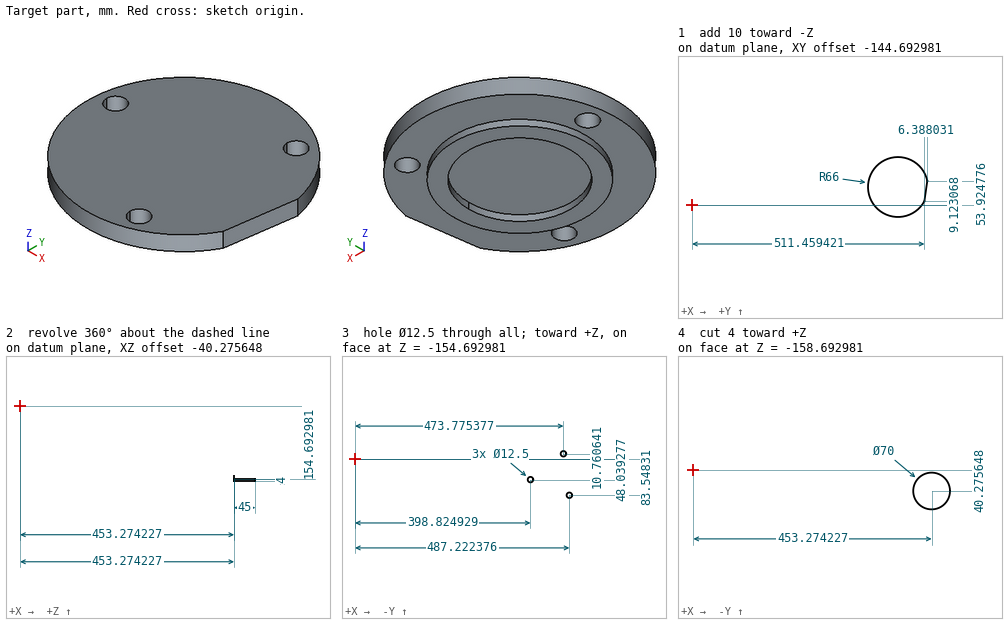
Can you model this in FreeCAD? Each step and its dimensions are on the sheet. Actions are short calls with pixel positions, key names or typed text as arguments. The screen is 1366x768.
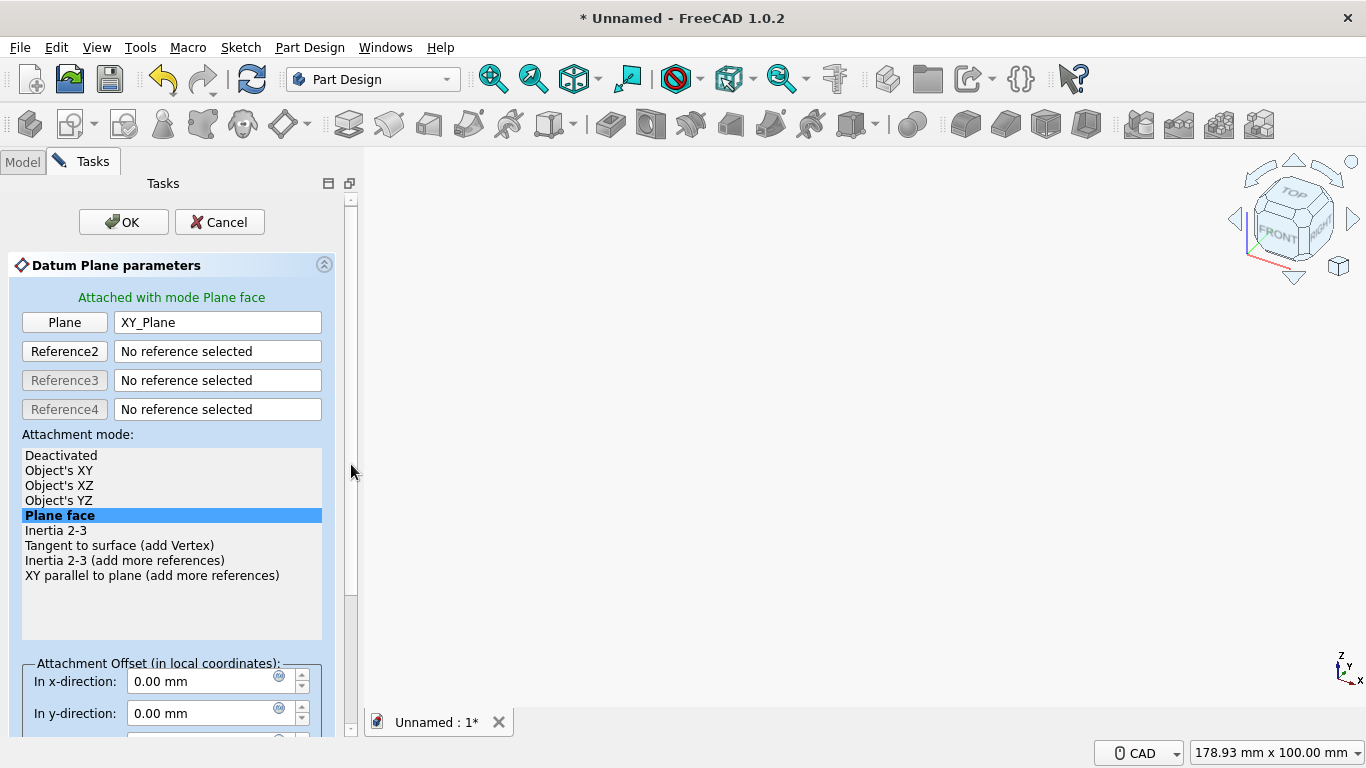
click(124, 222)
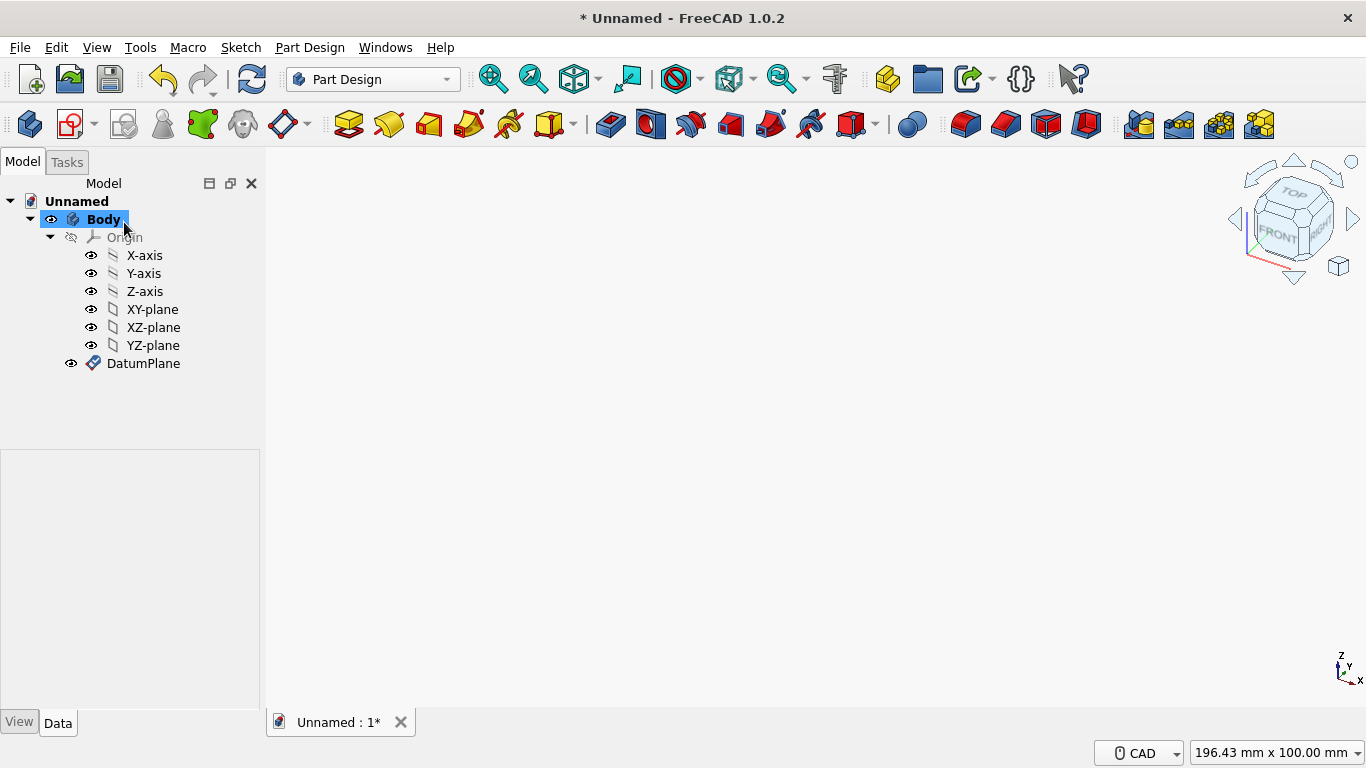
click(116, 363)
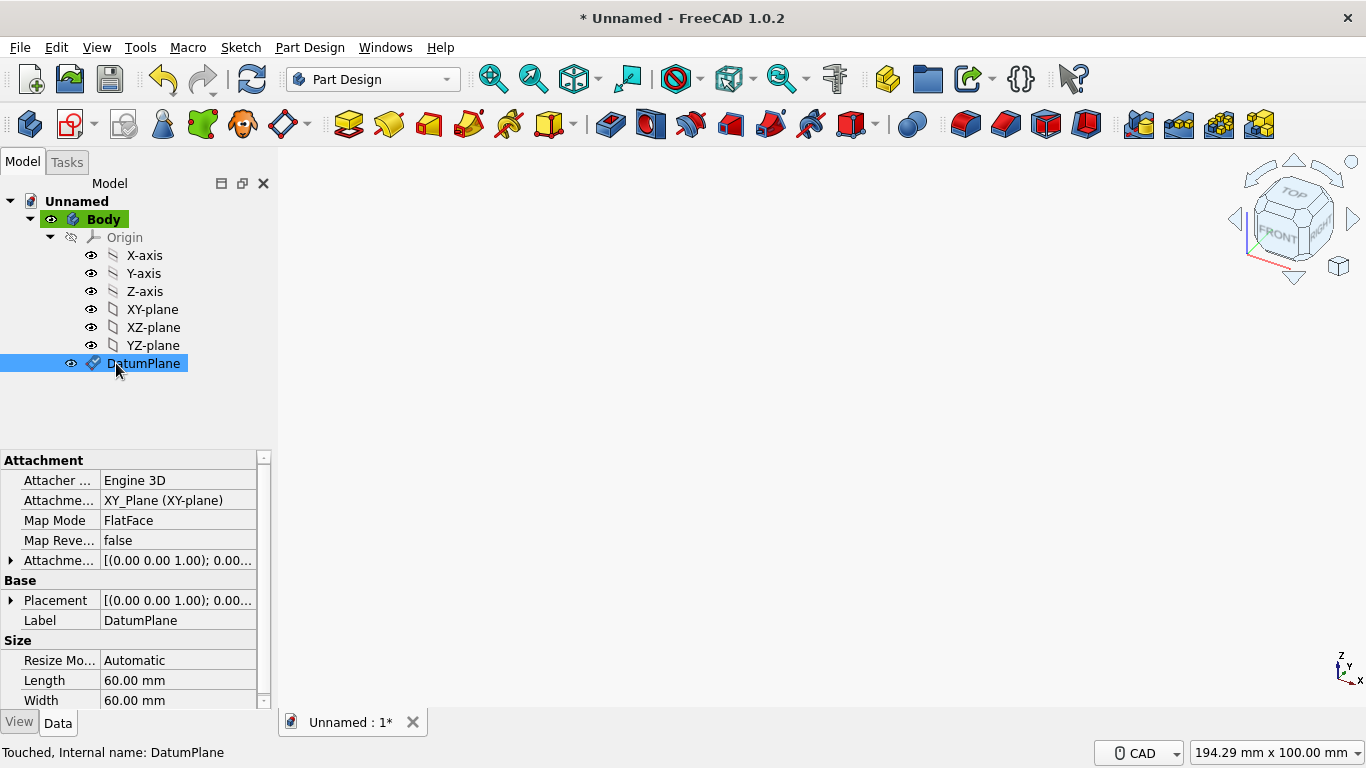
click(70, 124)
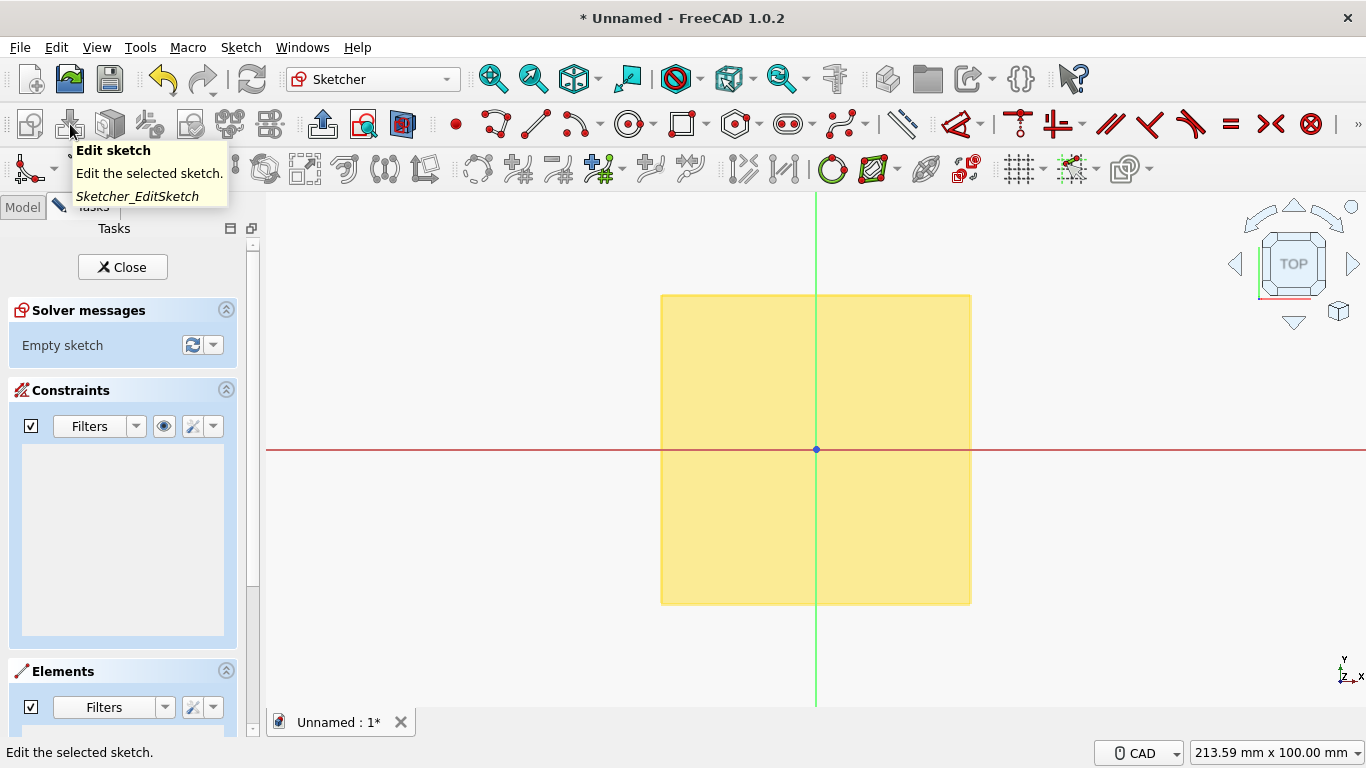
scroll(748, 450, down, 5)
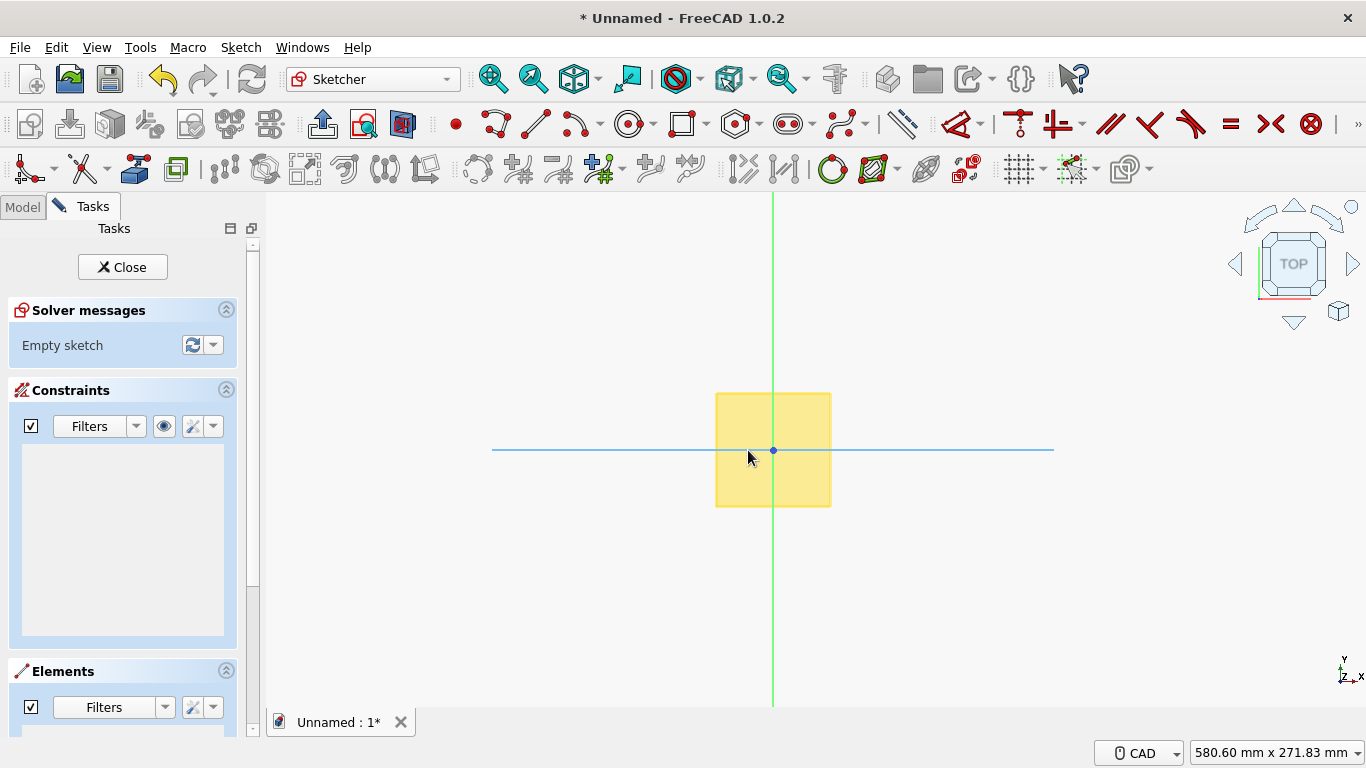
scroll(748, 450, down, 5)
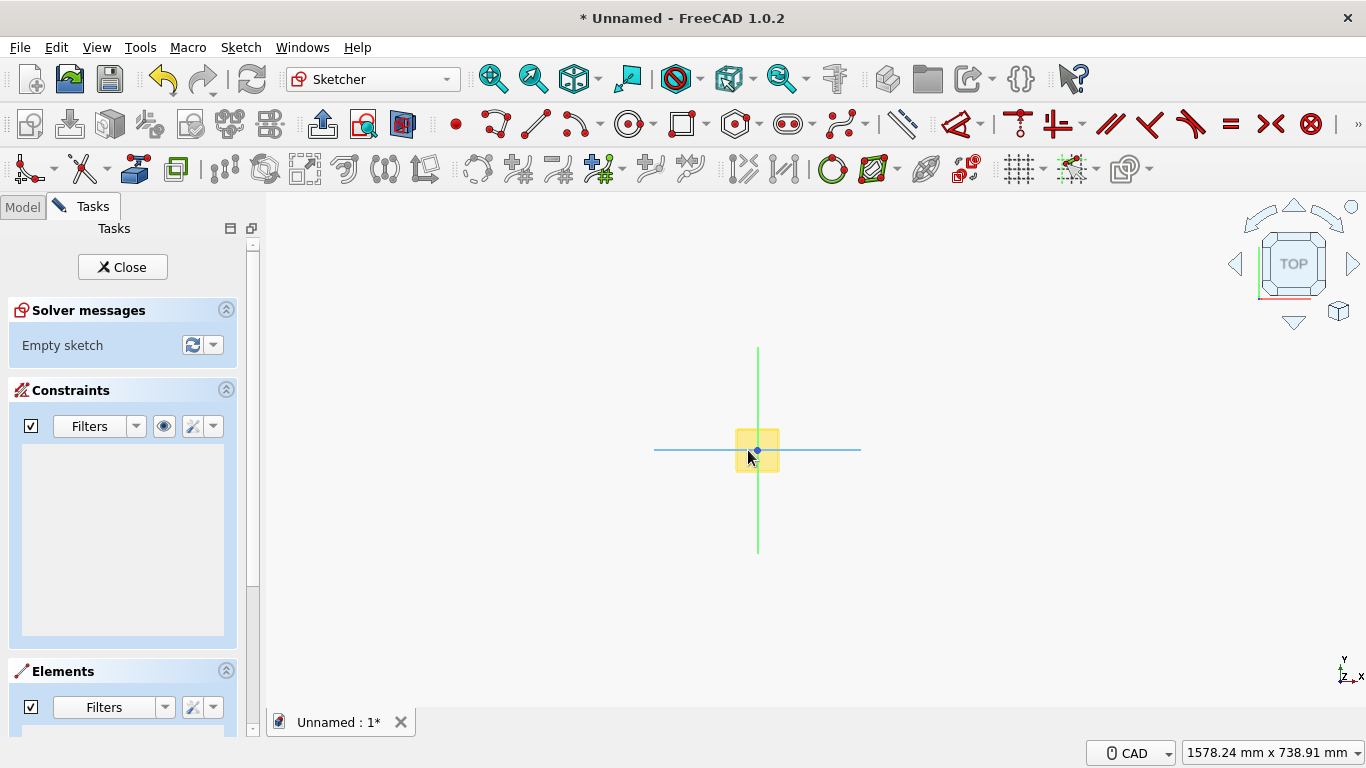
scroll(1124, 425, up, 10)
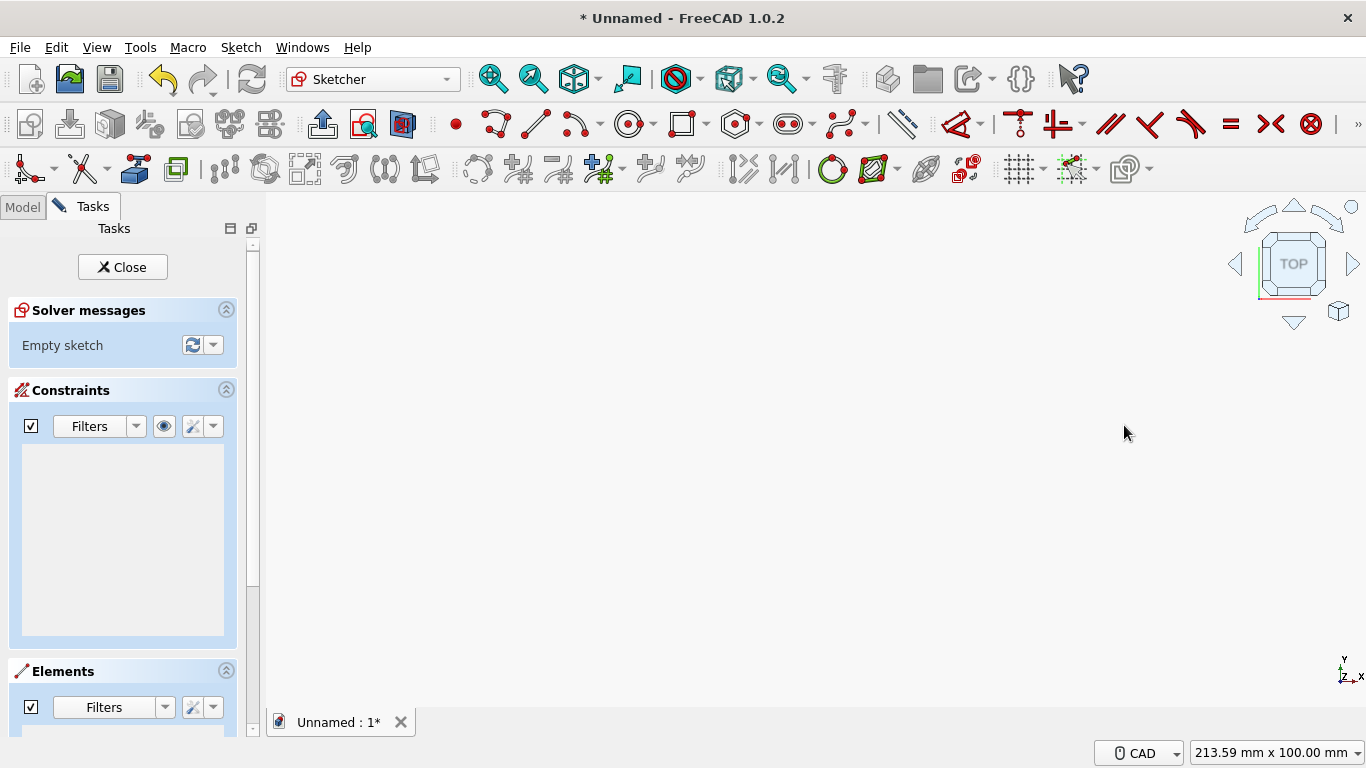
key(g)
key(l)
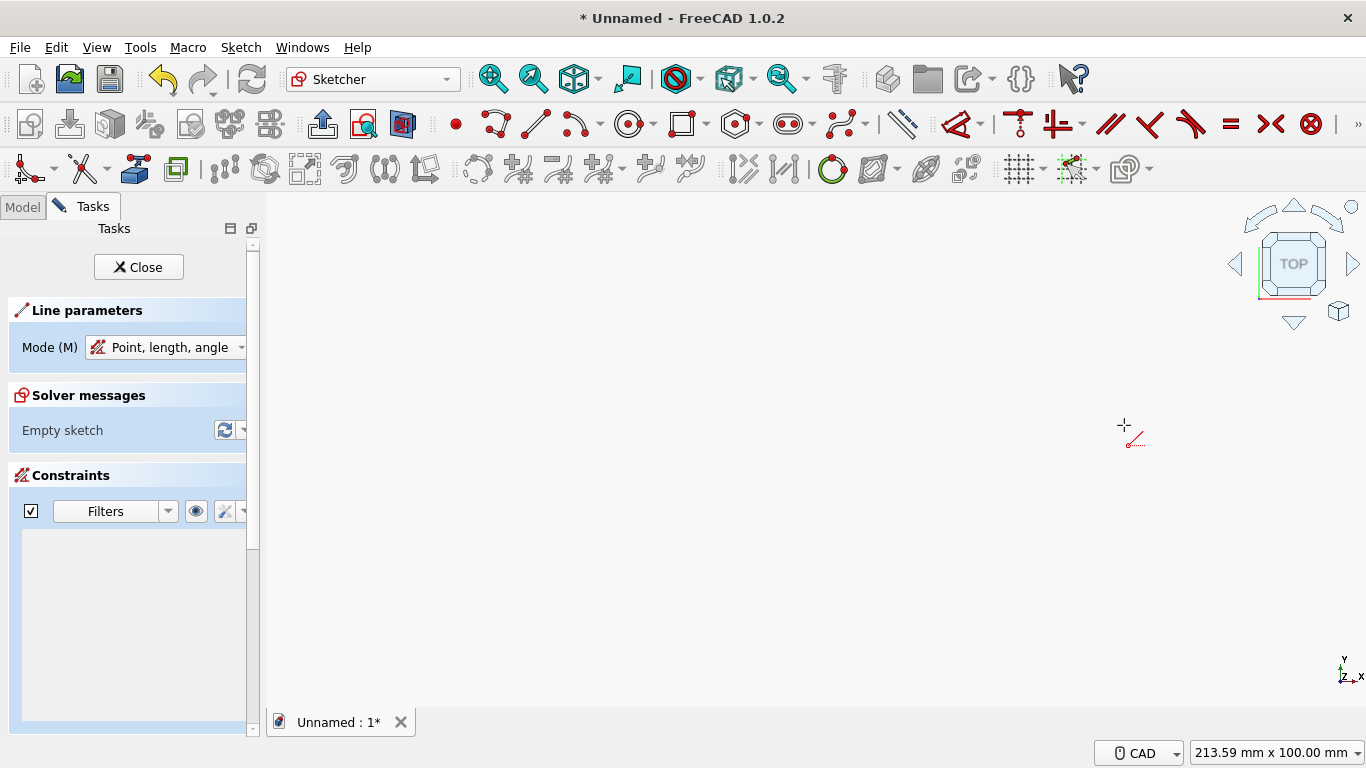
click(1046, 563)
click(1078, 332)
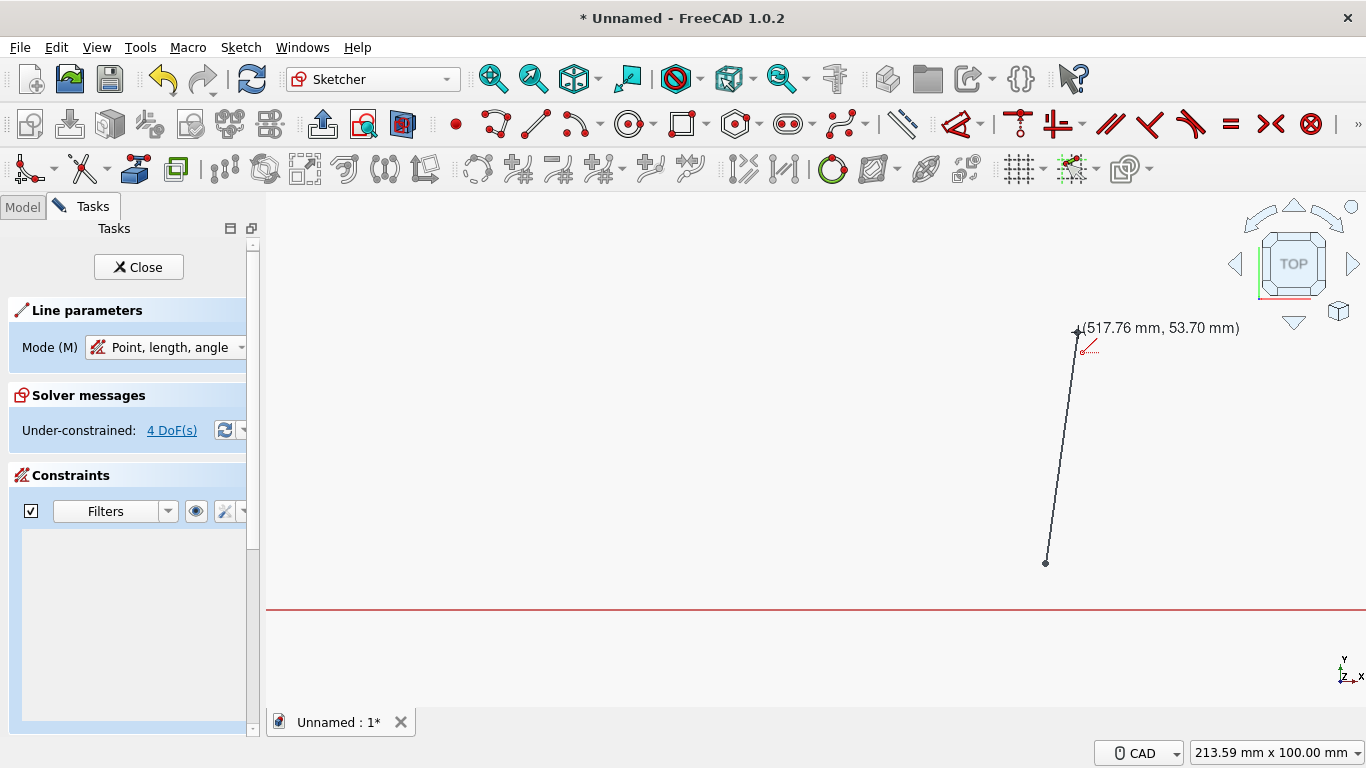
key(g)
key(3)
key(a)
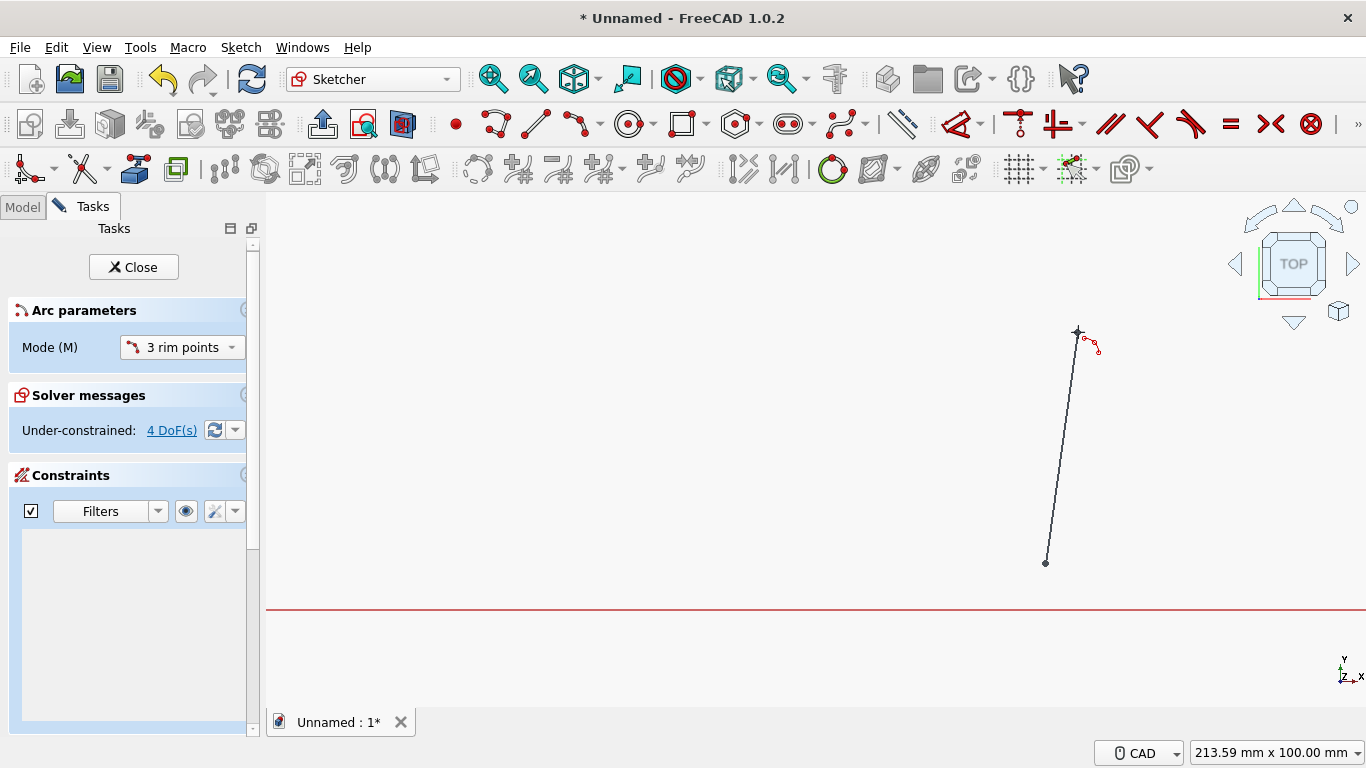
click(1078, 333)
click(1046, 564)
click(409, 354)
key(Escape)